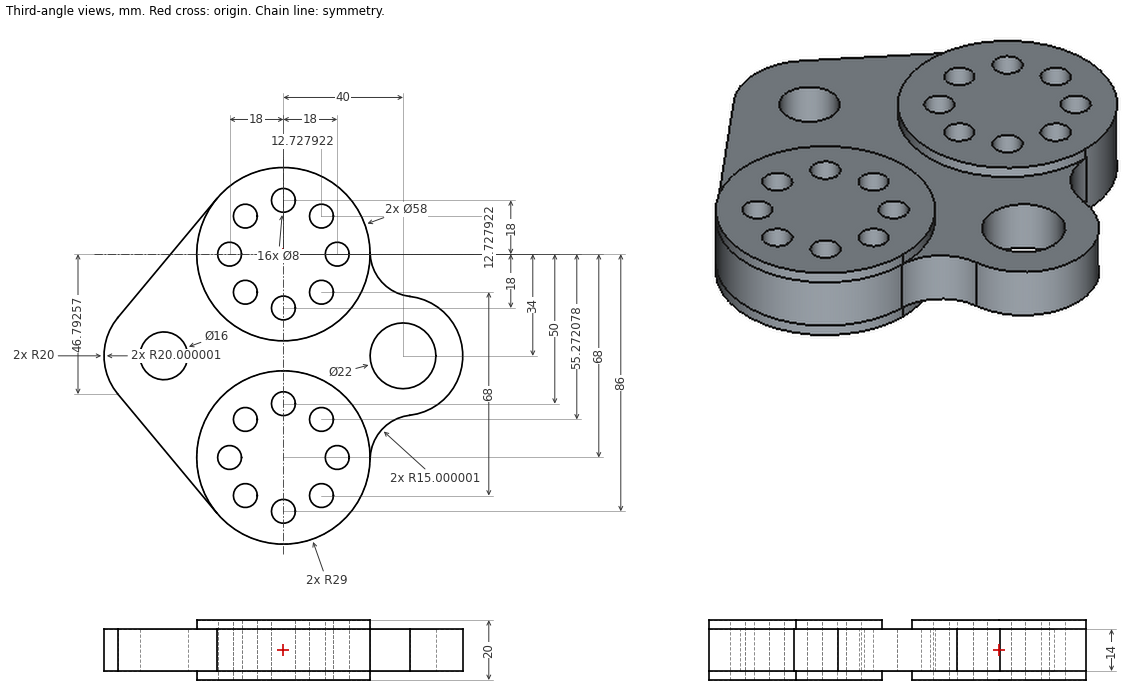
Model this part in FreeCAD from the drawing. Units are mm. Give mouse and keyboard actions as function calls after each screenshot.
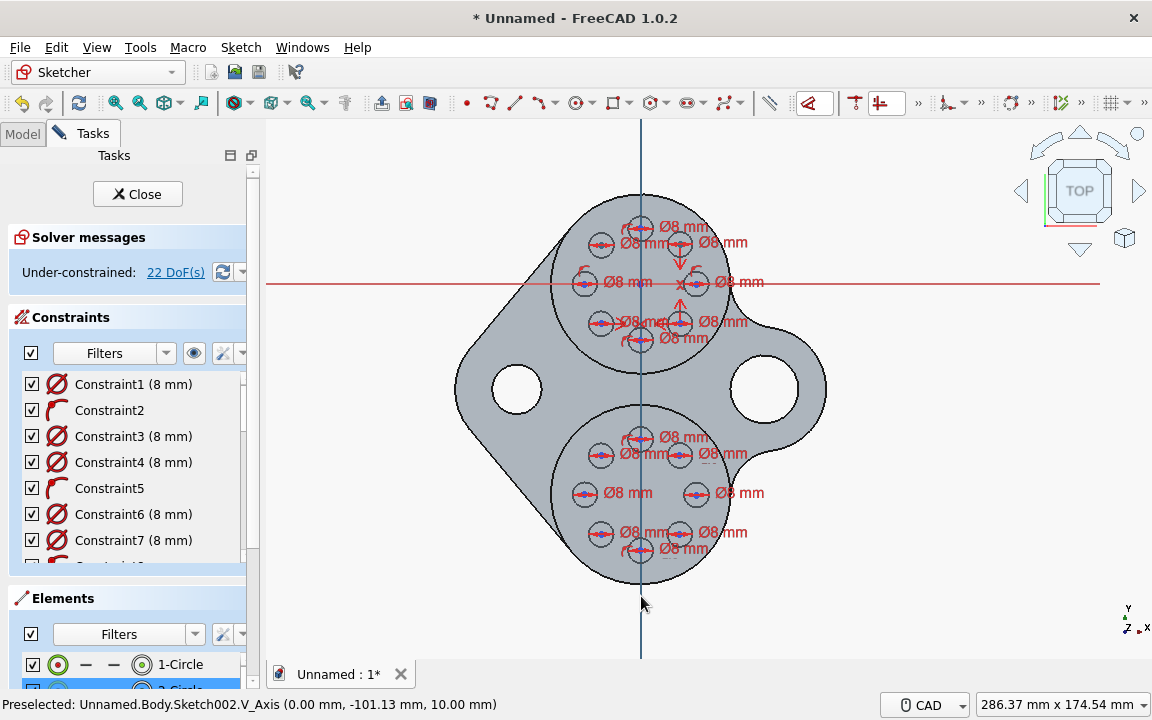
key(s)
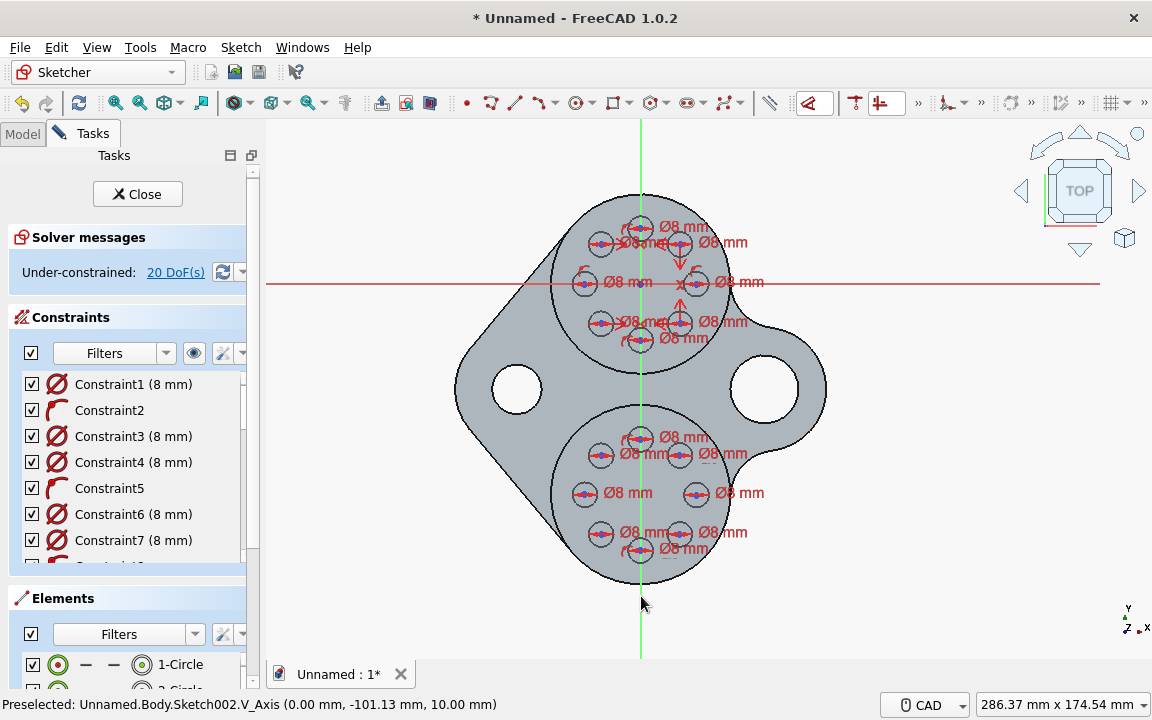
click(680, 534)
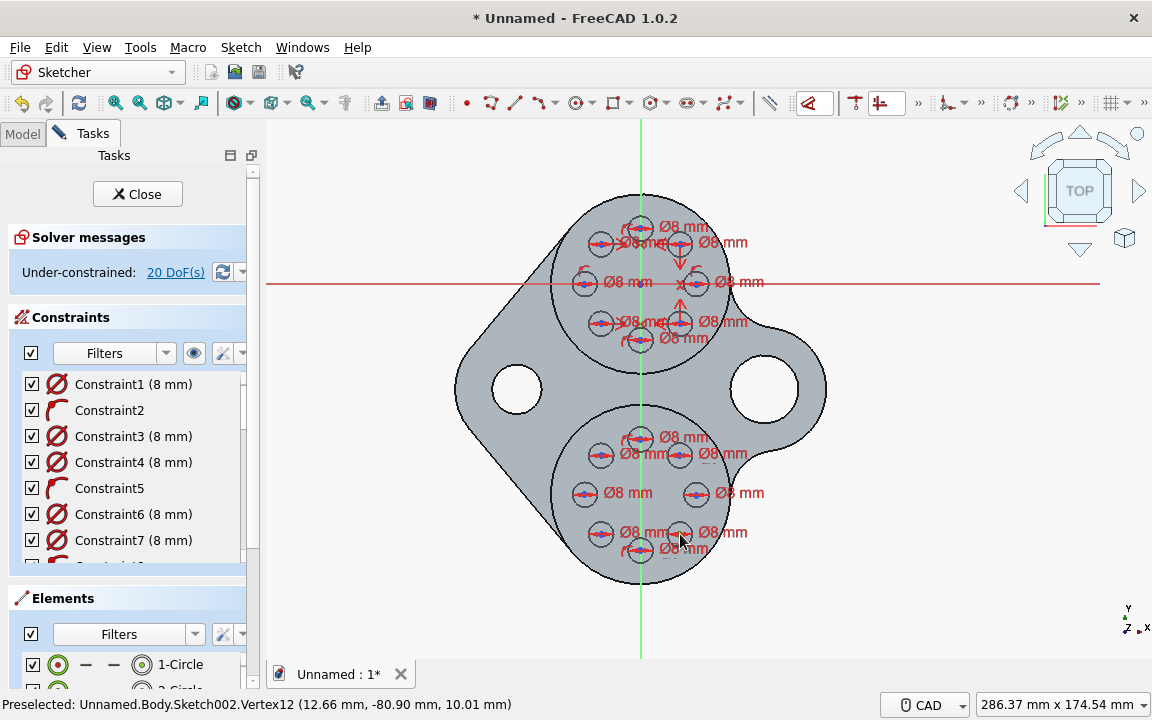
click(601, 534)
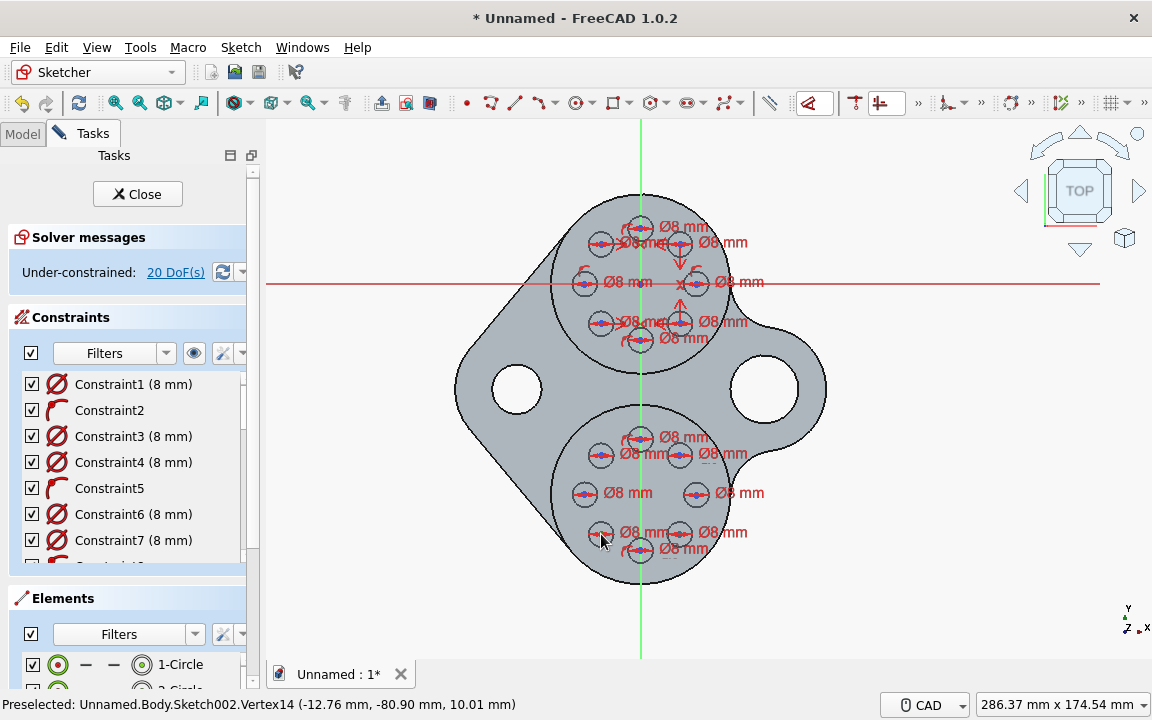
click(641, 596)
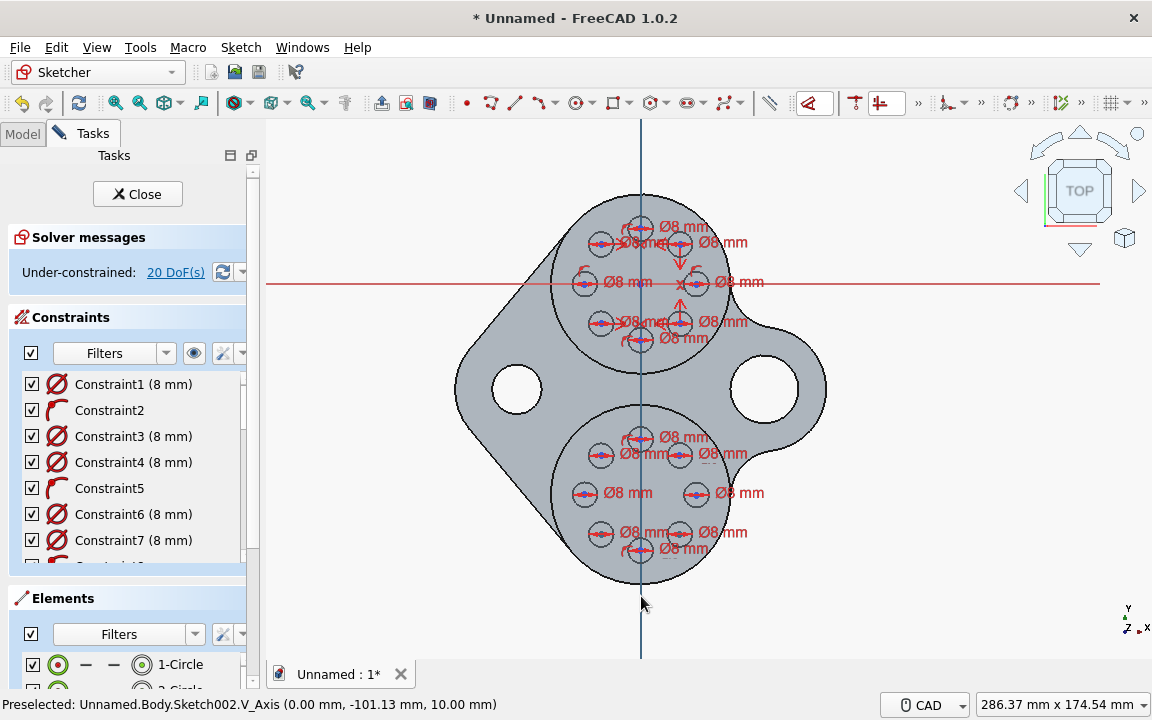
key(s)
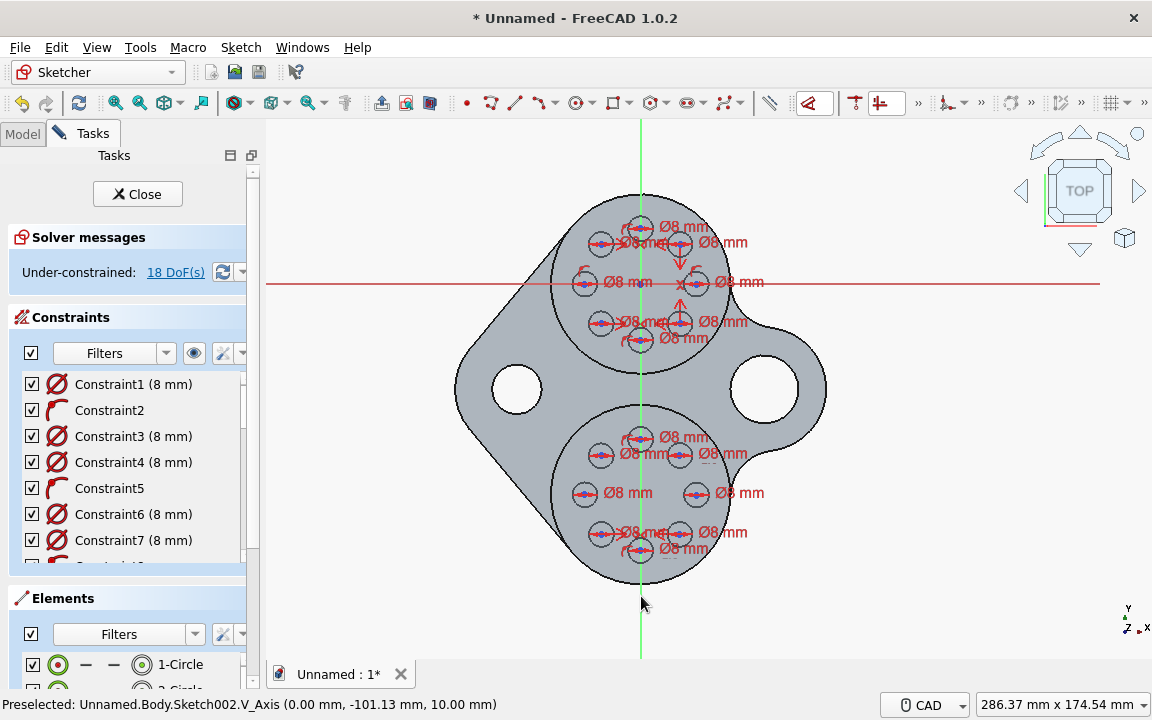
click(697, 495)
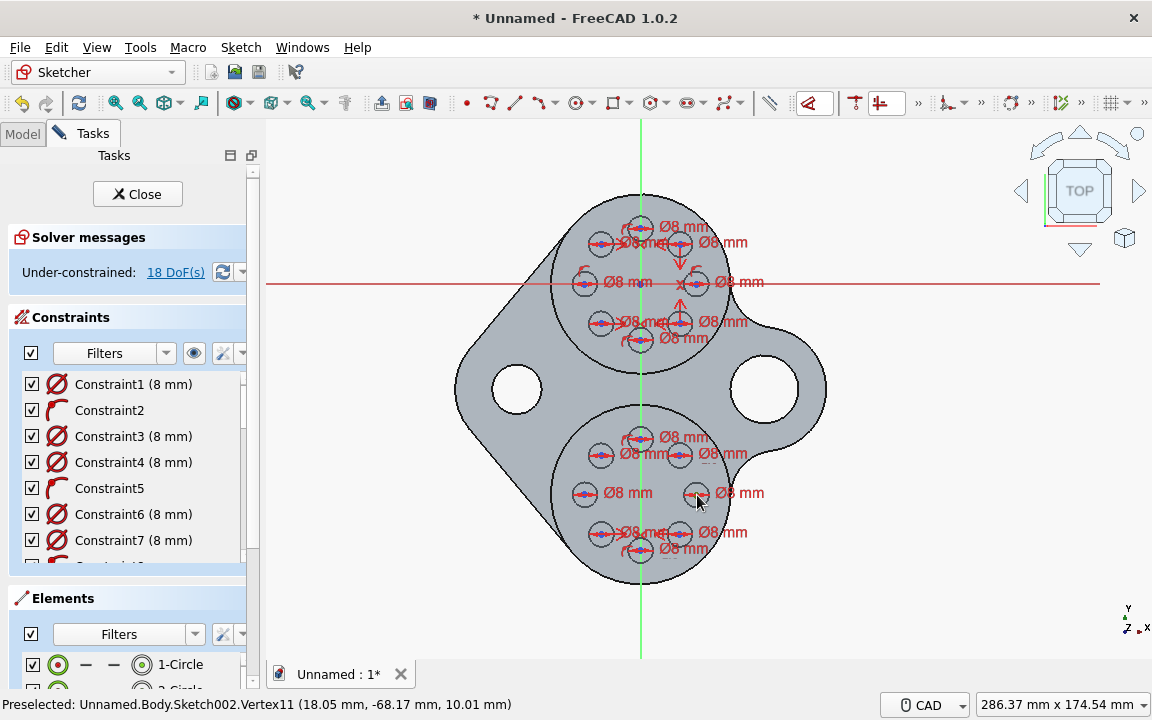
click(585, 495)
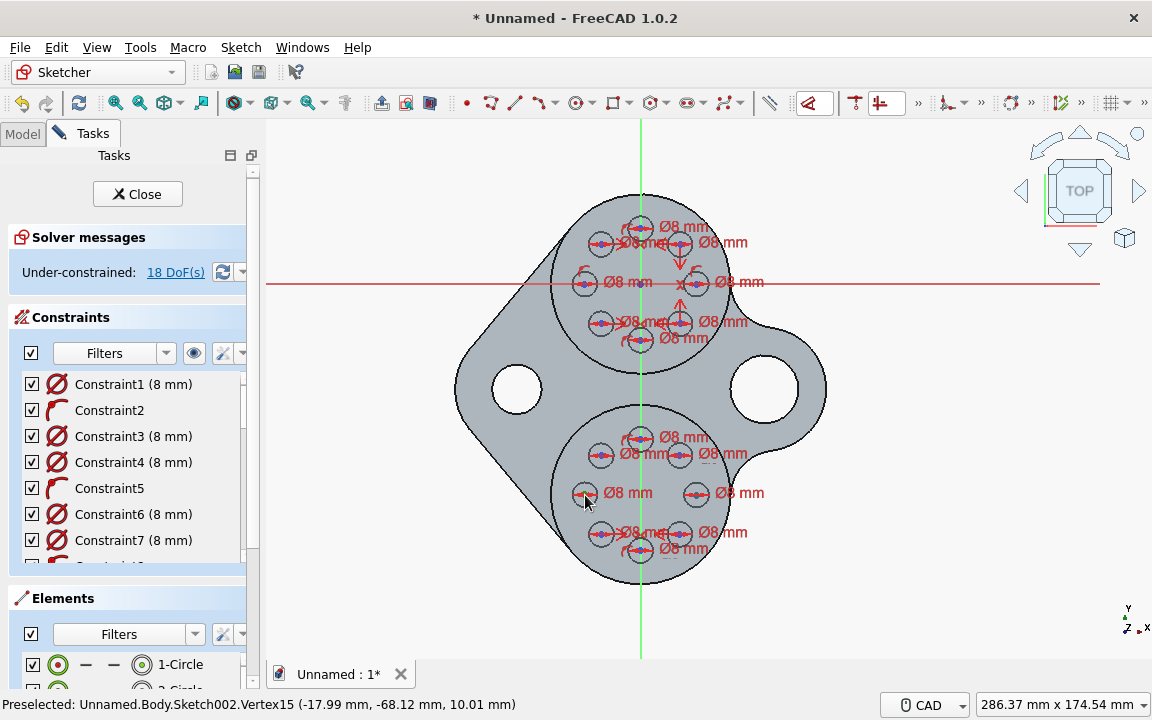
click(641, 596)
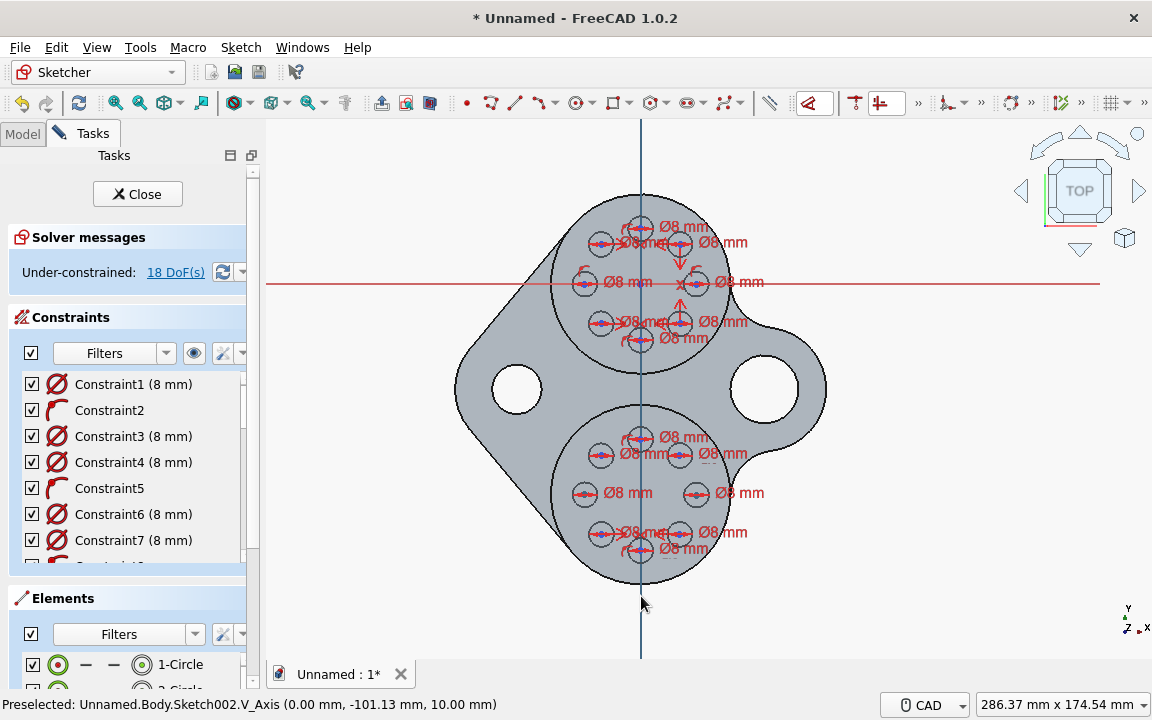
key(s)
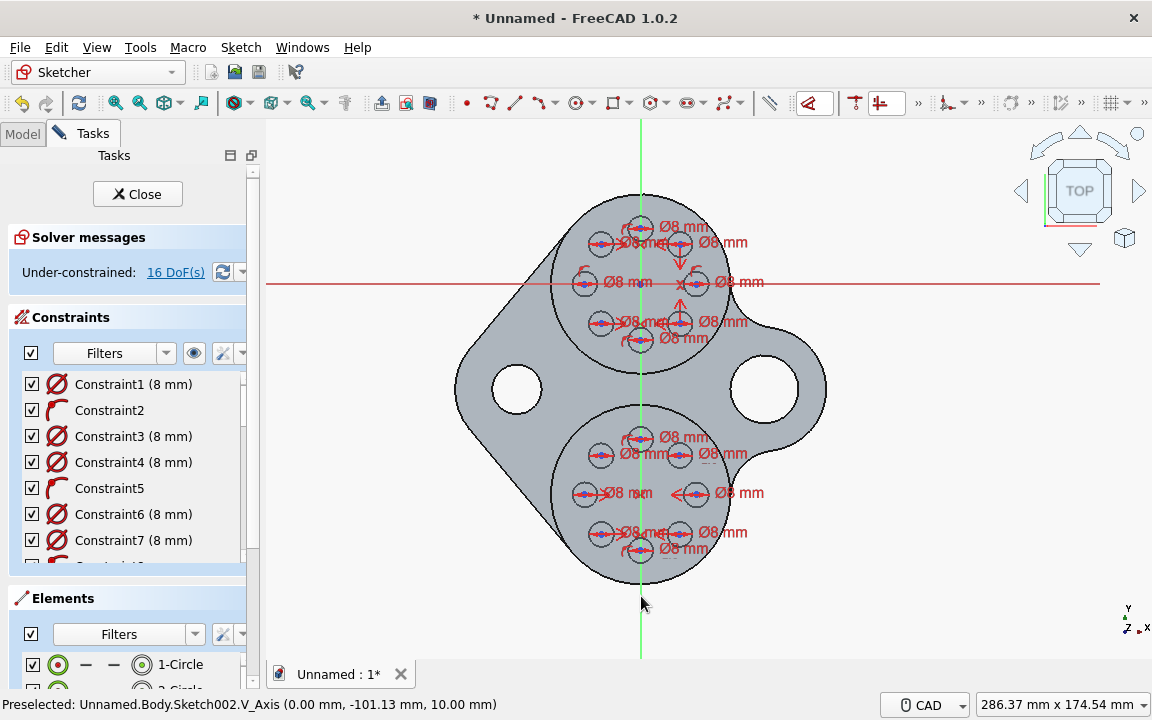
click(680, 456)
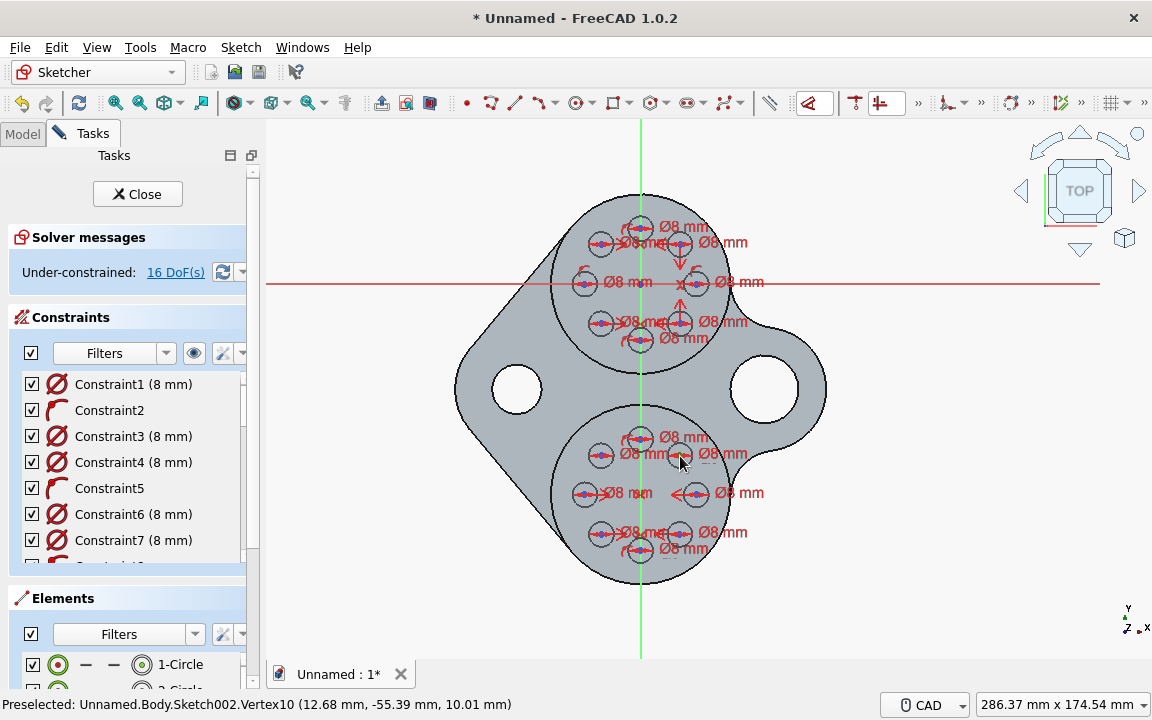
click(601, 456)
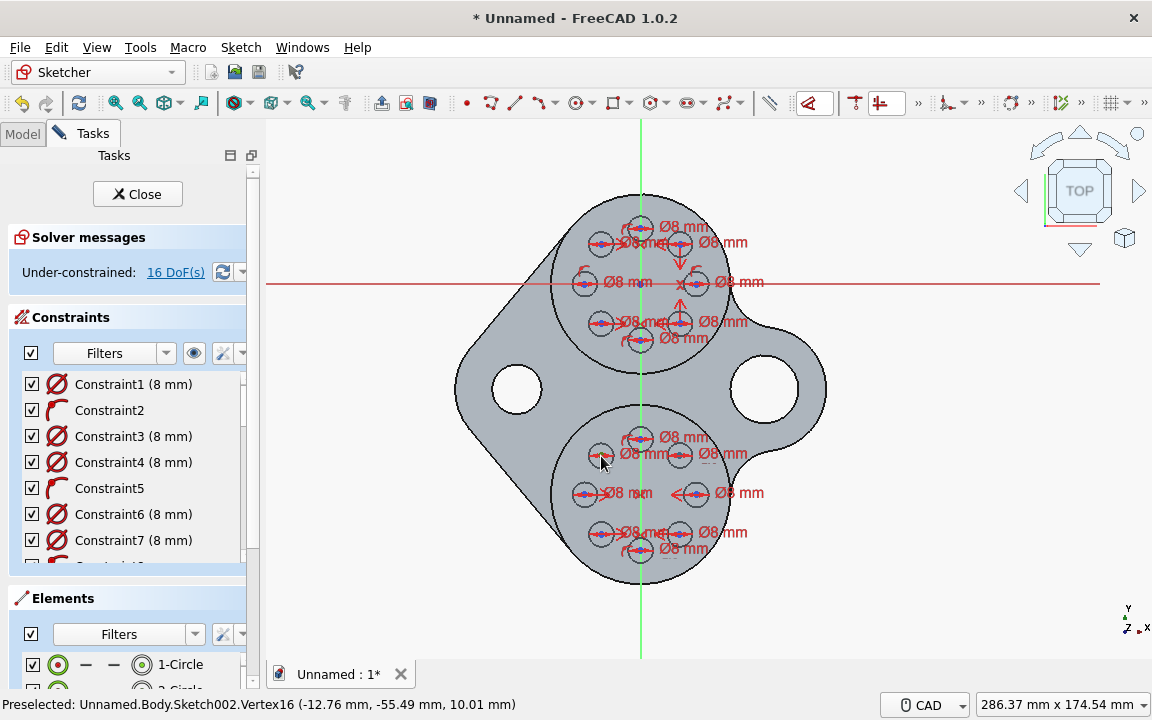
click(641, 596)